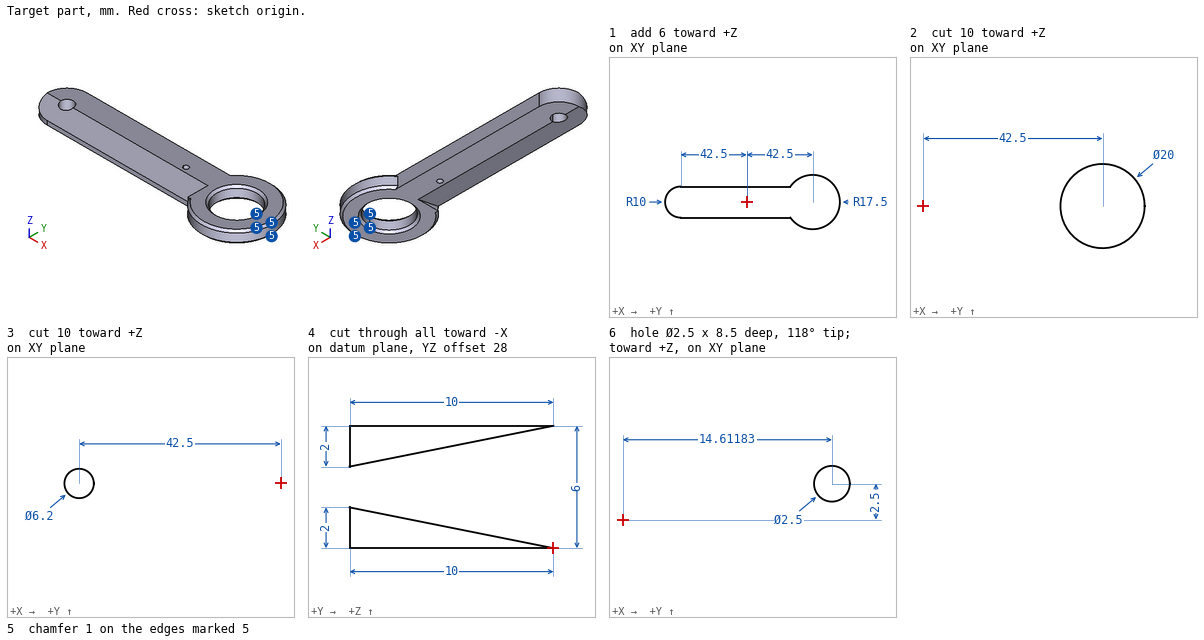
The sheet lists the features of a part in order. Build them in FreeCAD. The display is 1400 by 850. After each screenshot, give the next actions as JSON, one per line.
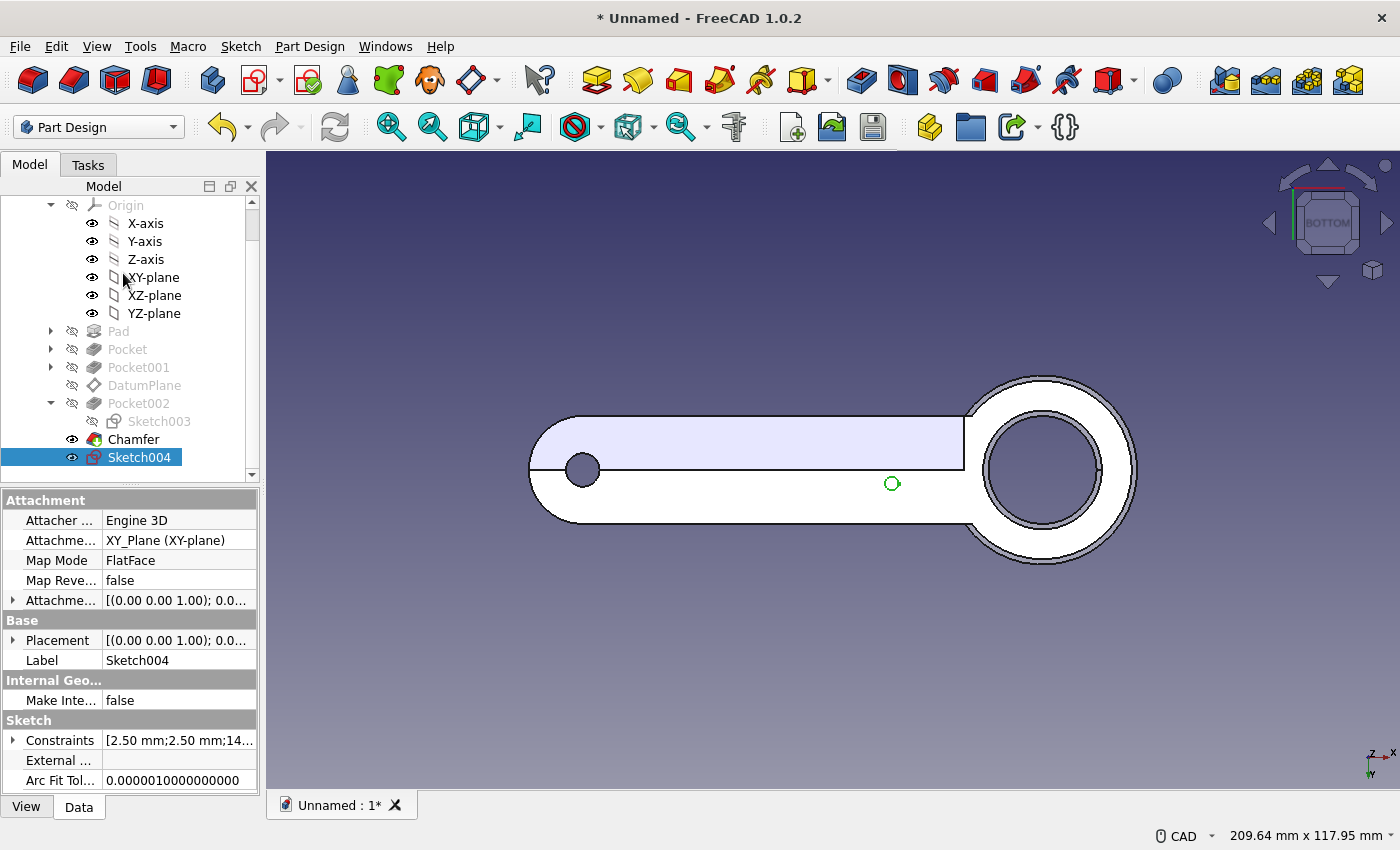
{"action": "left_click", "coordinate": [903, 80]}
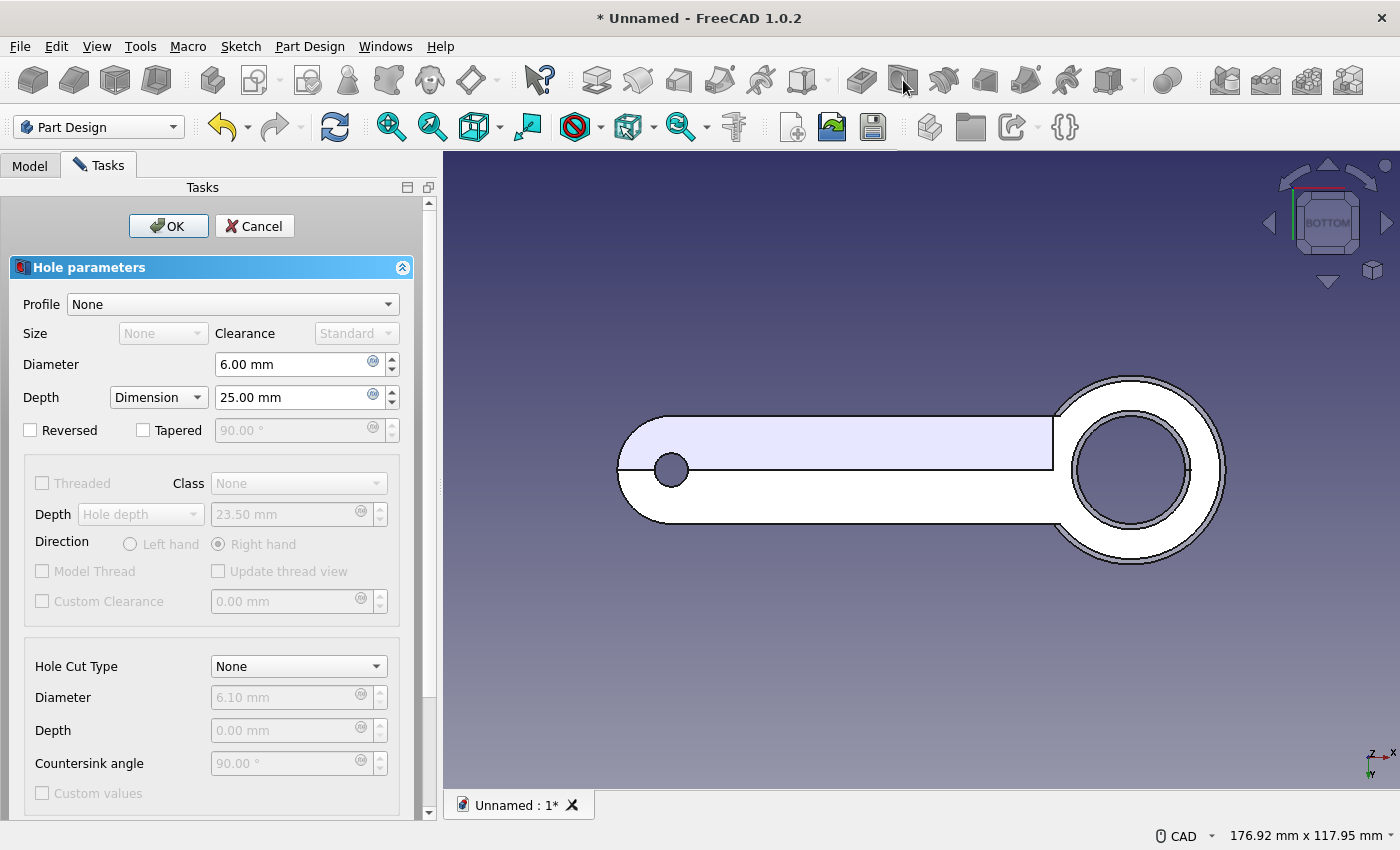
{"action": "triple_click", "coordinate": [300, 364]}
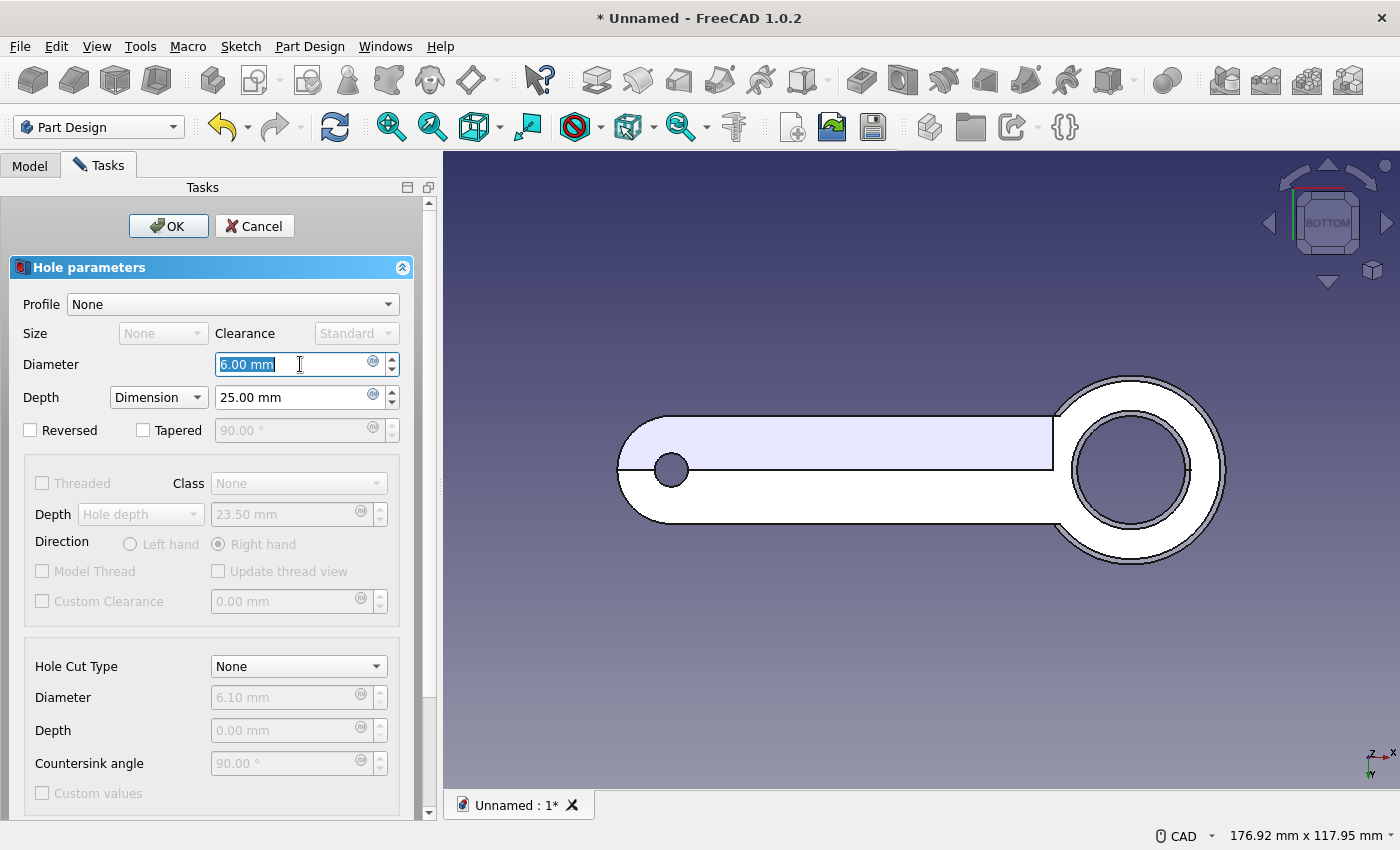
{"action": "type", "text": "2.5"}
{"action": "key", "text": "Tab"}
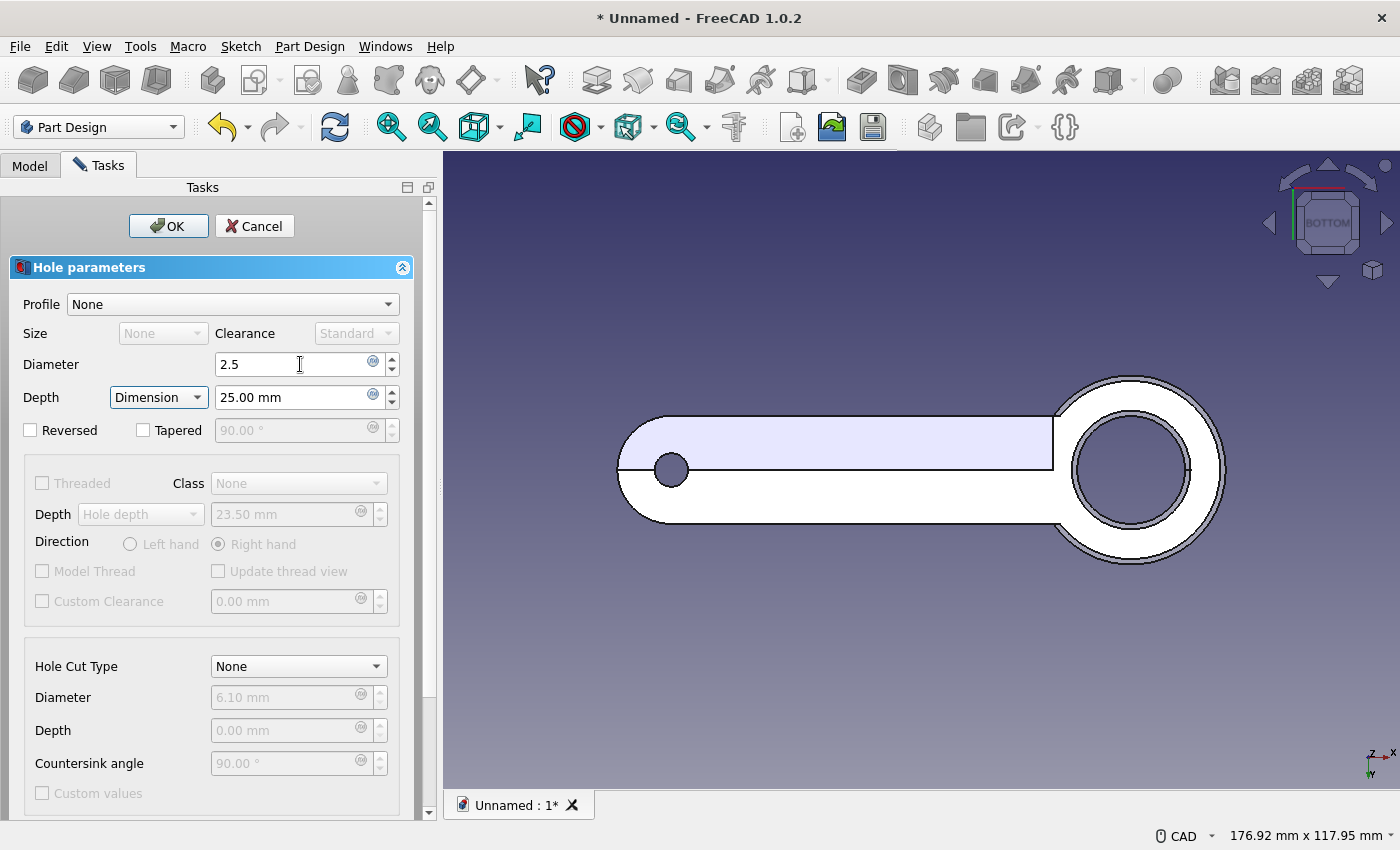
{"action": "triple_click", "coordinate": [300, 398]}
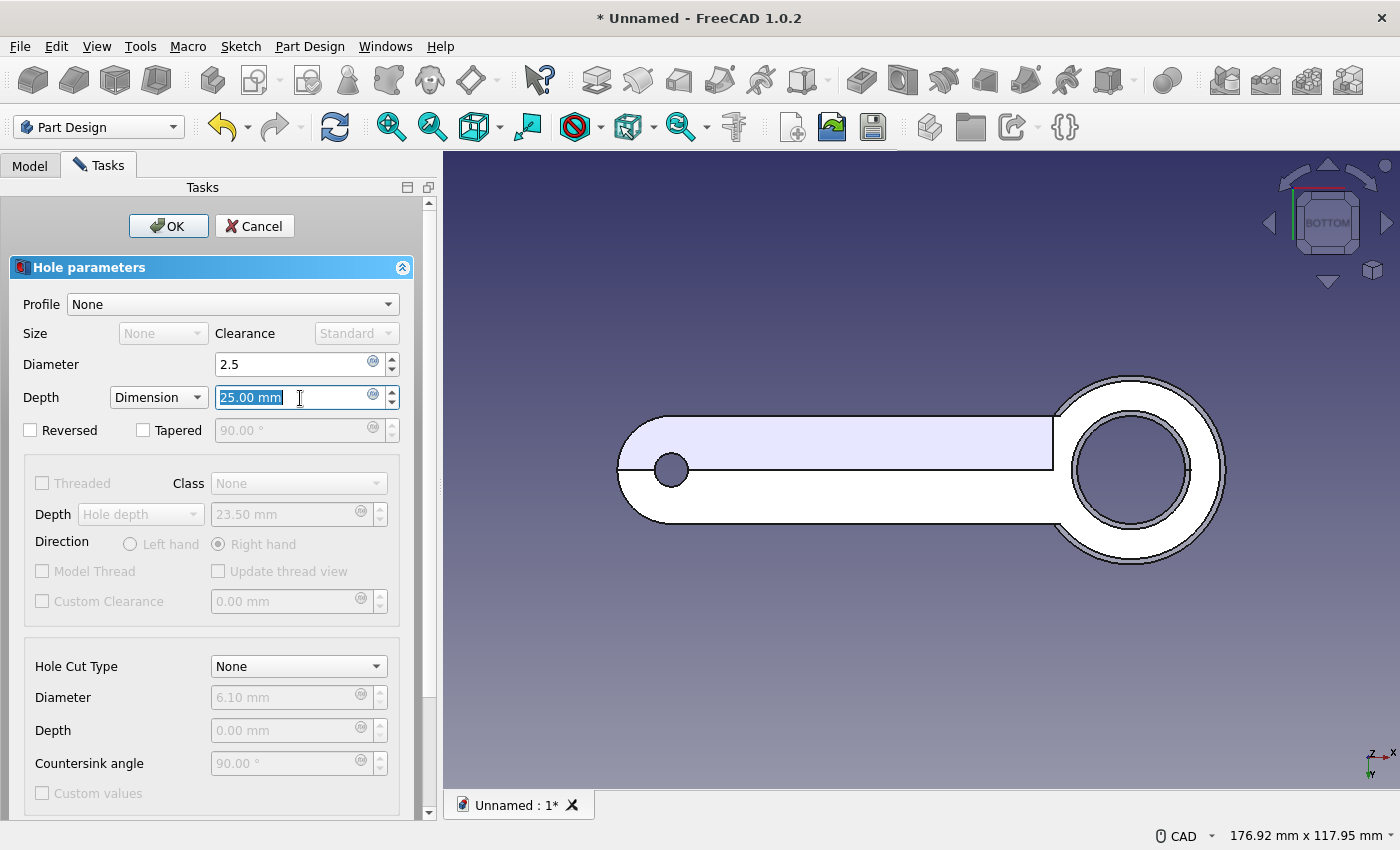
{"action": "type", "text": "8.5"}
{"action": "key", "text": "Tab"}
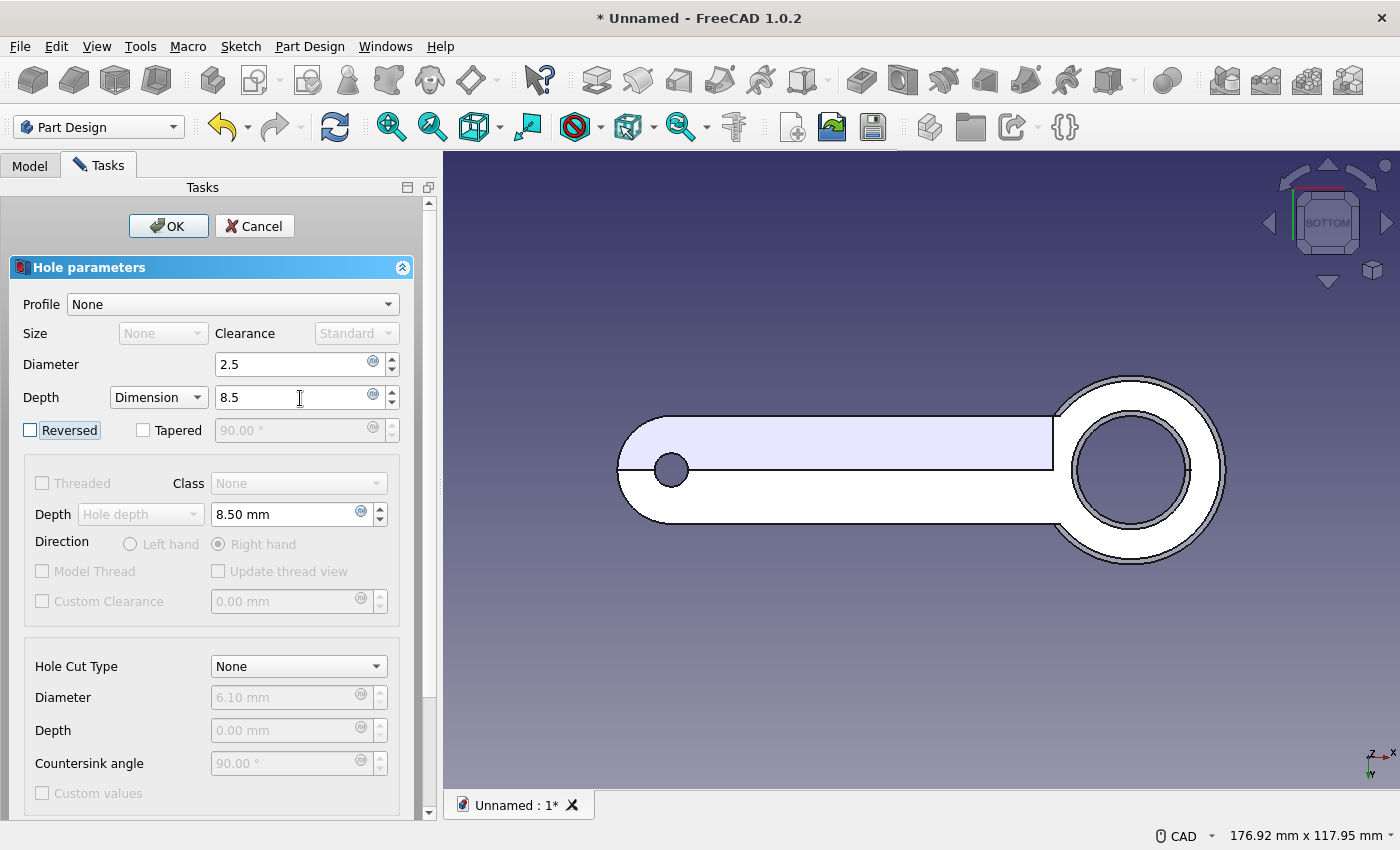
{"action": "left_click", "coordinate": [31, 430]}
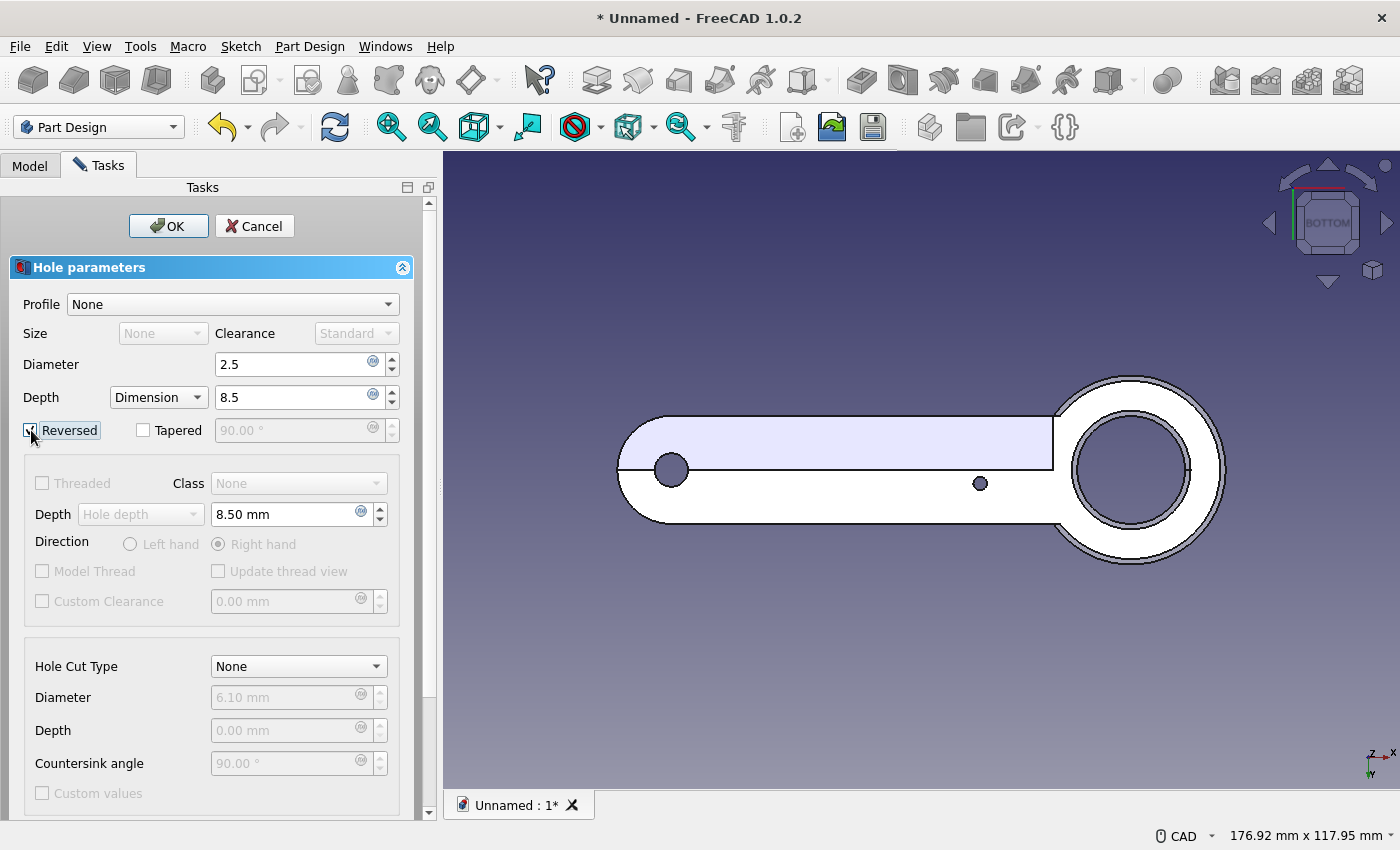
{"action": "left_click", "coordinate": [169, 226]}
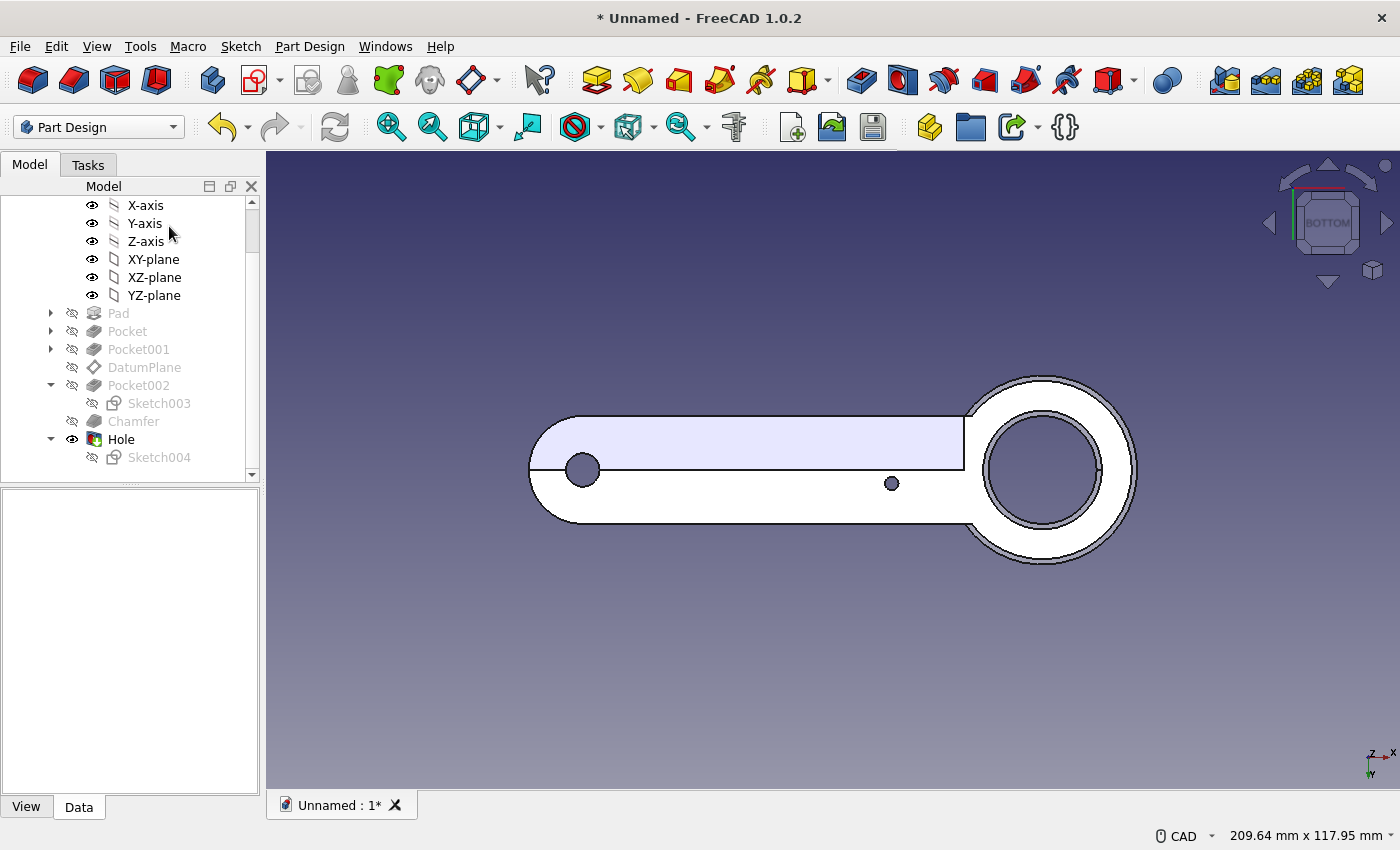
{"action": "key", "text": "0"}